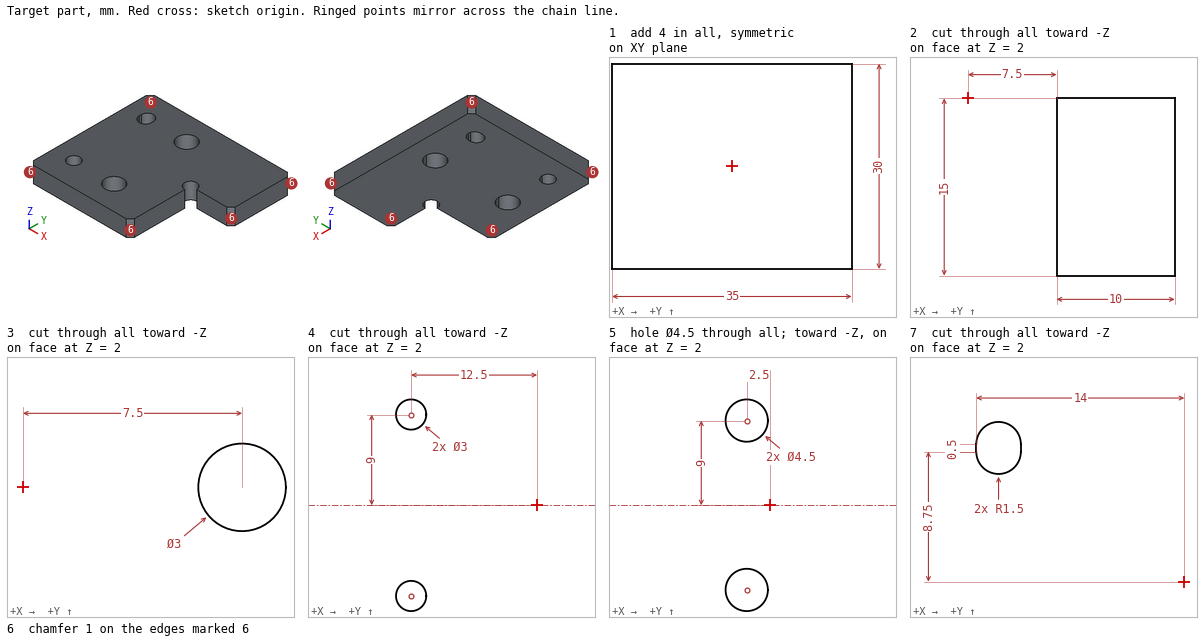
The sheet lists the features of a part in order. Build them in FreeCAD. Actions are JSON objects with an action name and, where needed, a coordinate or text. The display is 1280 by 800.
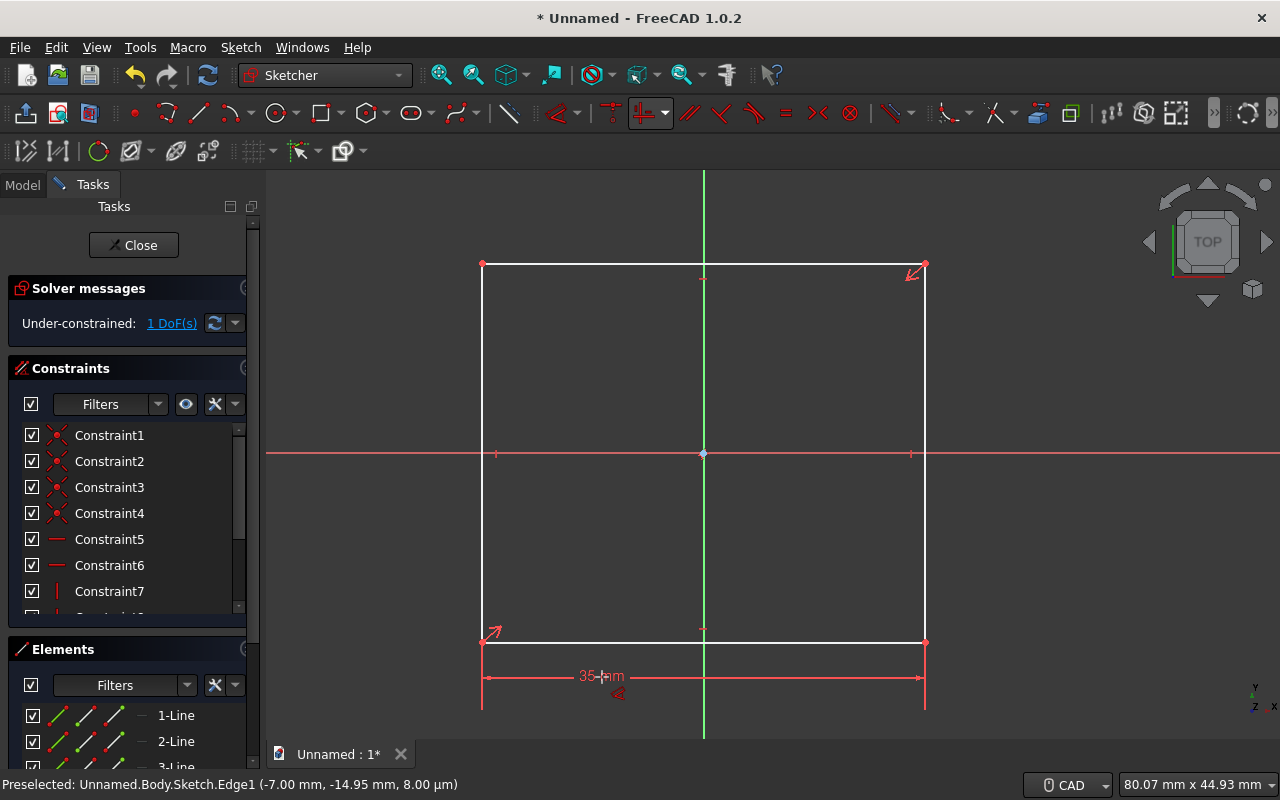
{"action": "left_click", "coordinate": [925, 529]}
{"action": "left_click", "coordinate": [959, 366]}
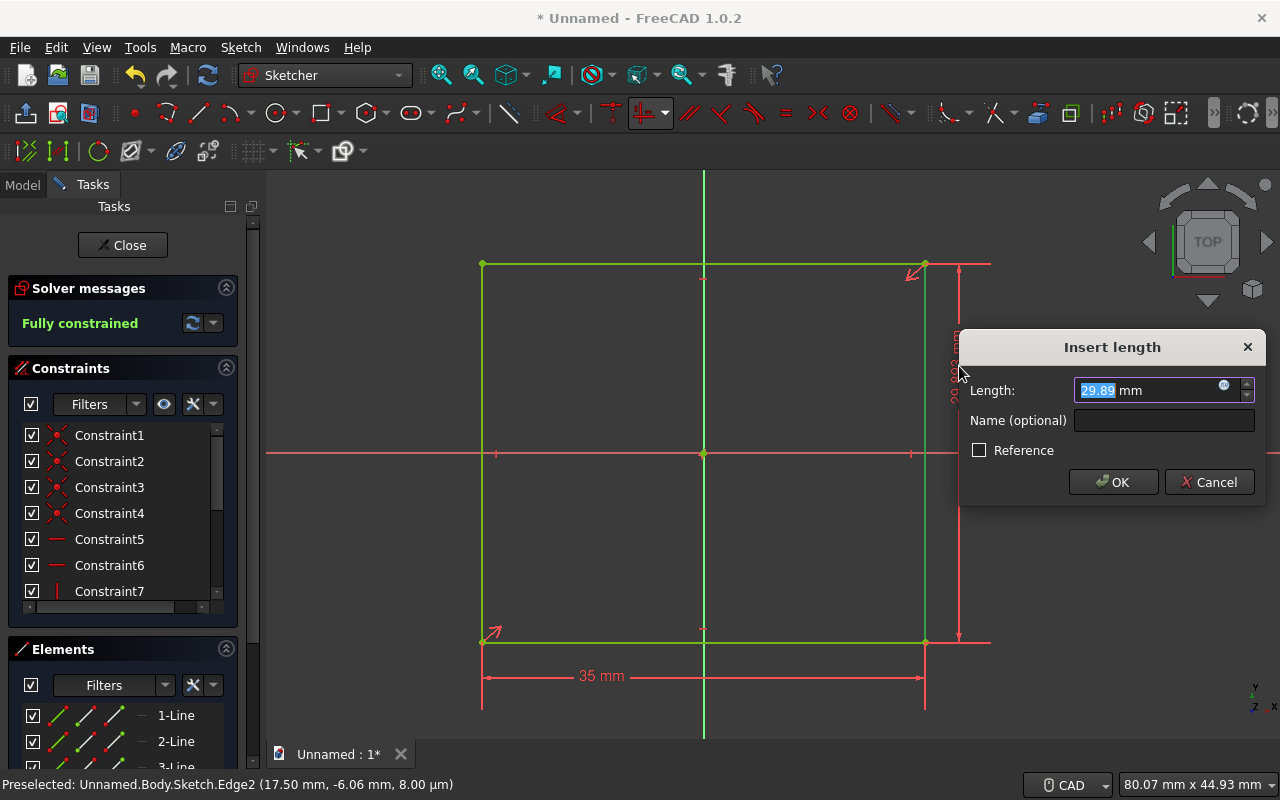
{"action": "type", "text": "30"}
{"action": "key", "text": "Return"}
{"action": "key", "text": "Escape"}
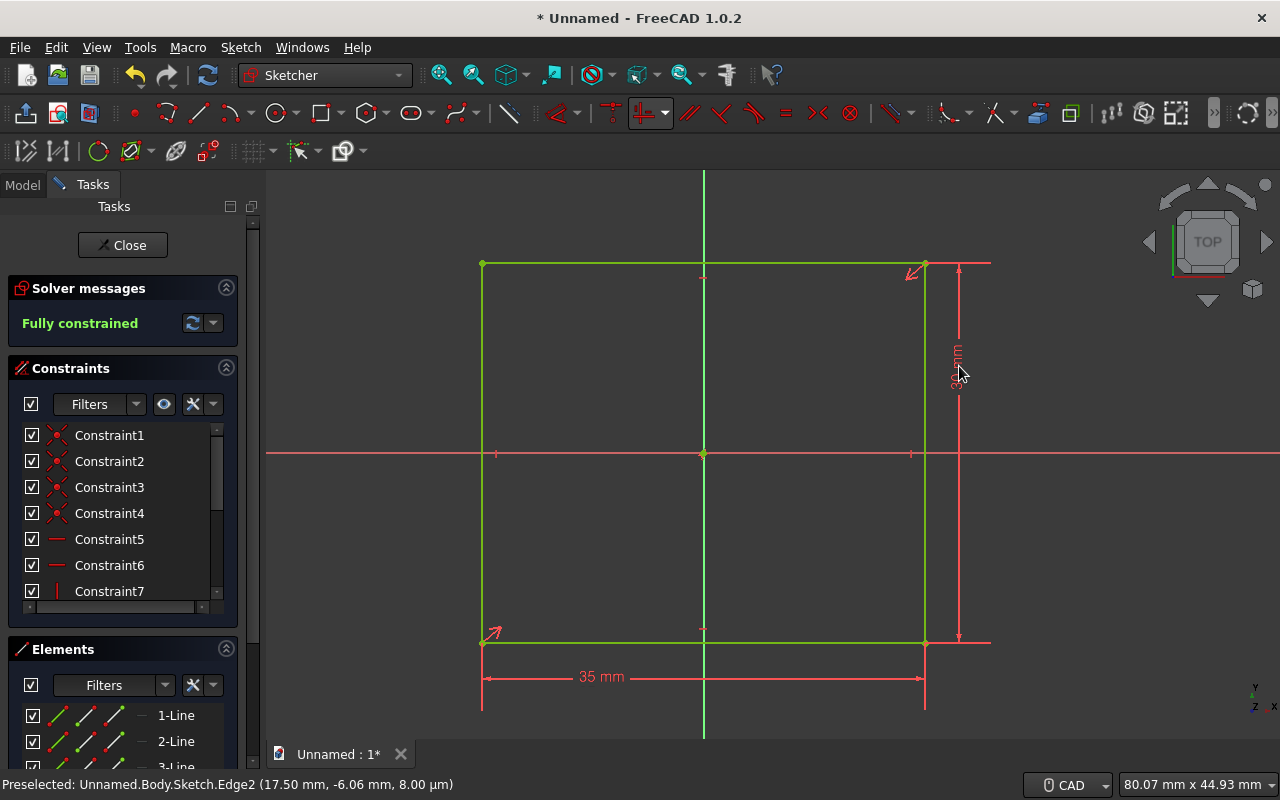
{"action": "left_click", "coordinate": [123, 245]}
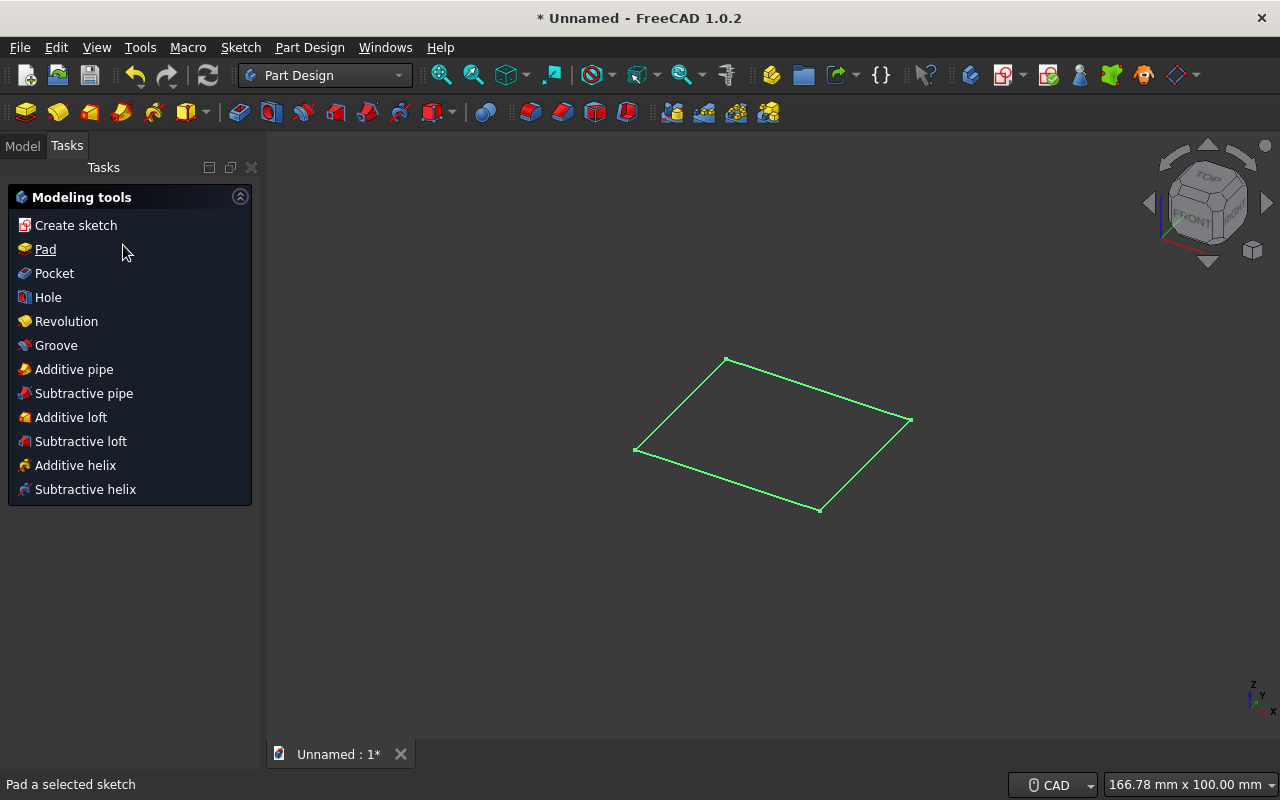
{"action": "left_click", "coordinate": [26, 112]}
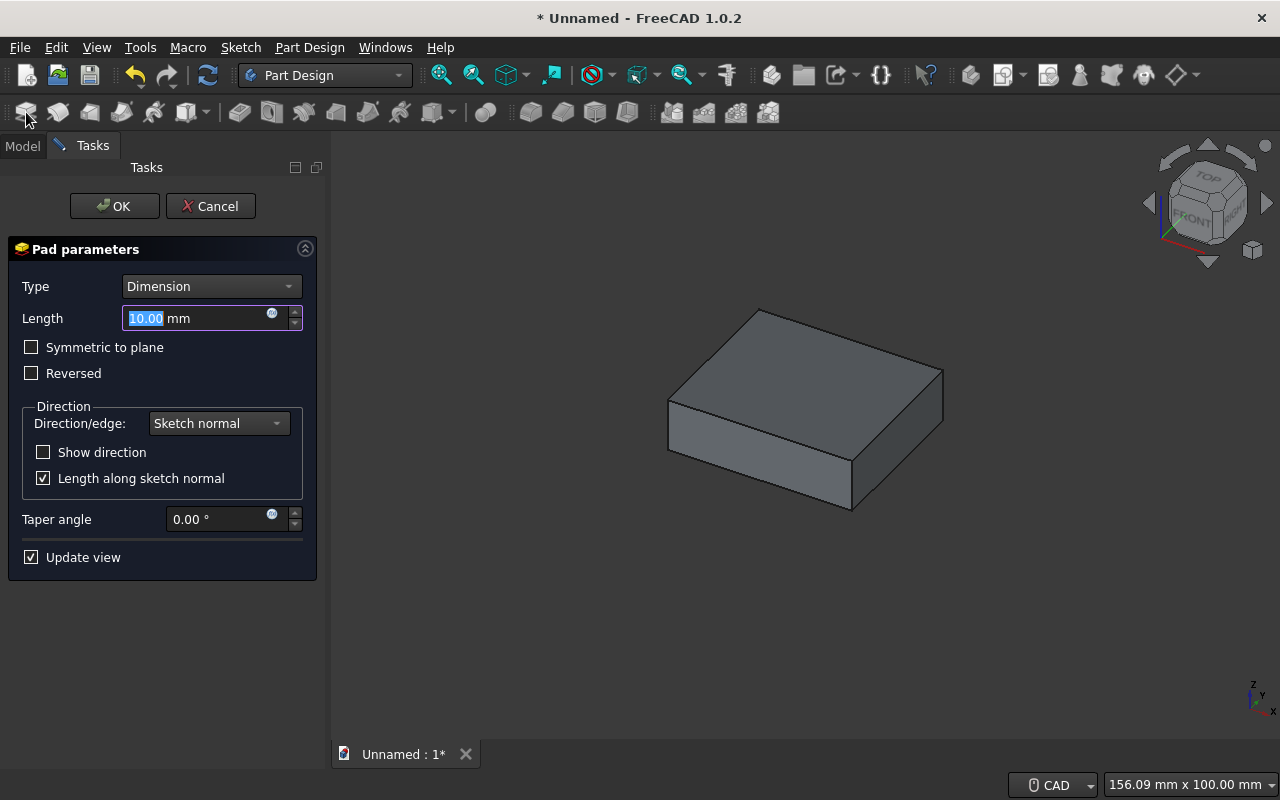
{"action": "type", "text": "4"}
{"action": "key", "text": "Tab"}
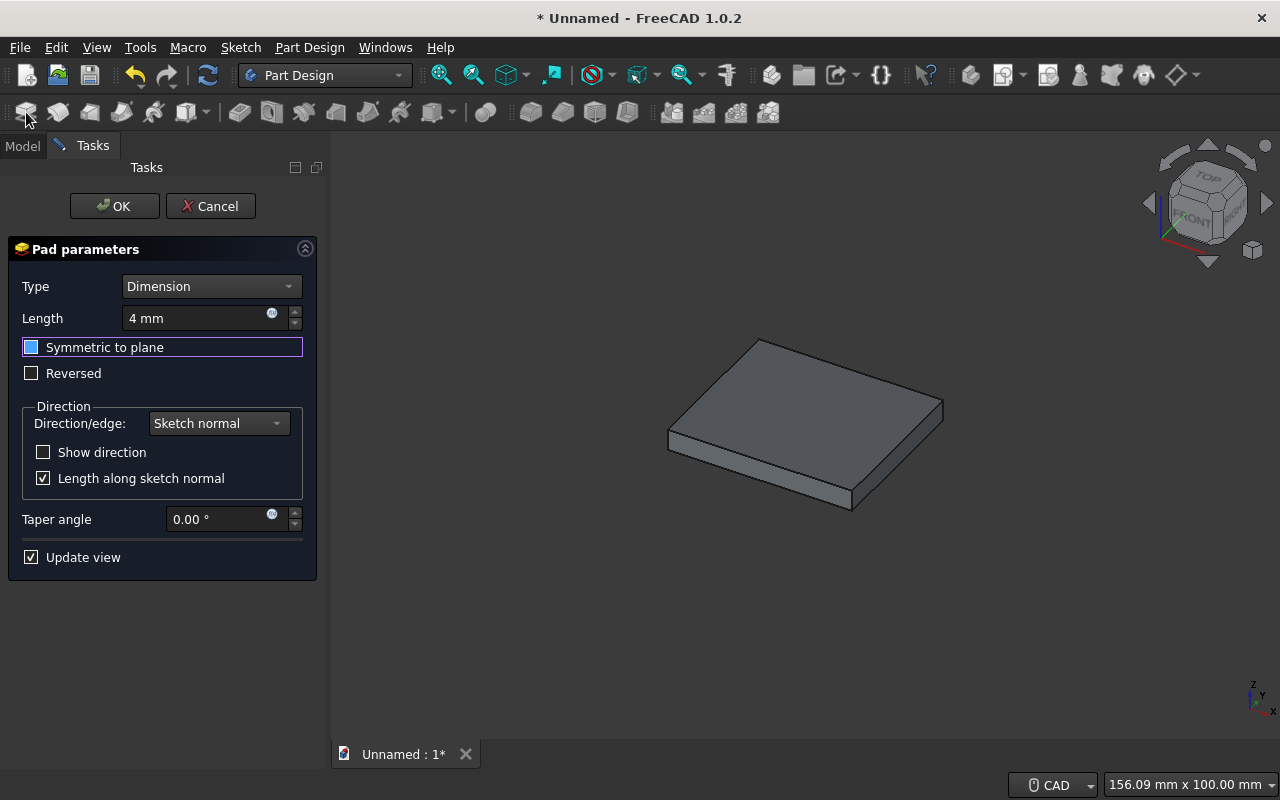
{"action": "left_click", "coordinate": [30, 347]}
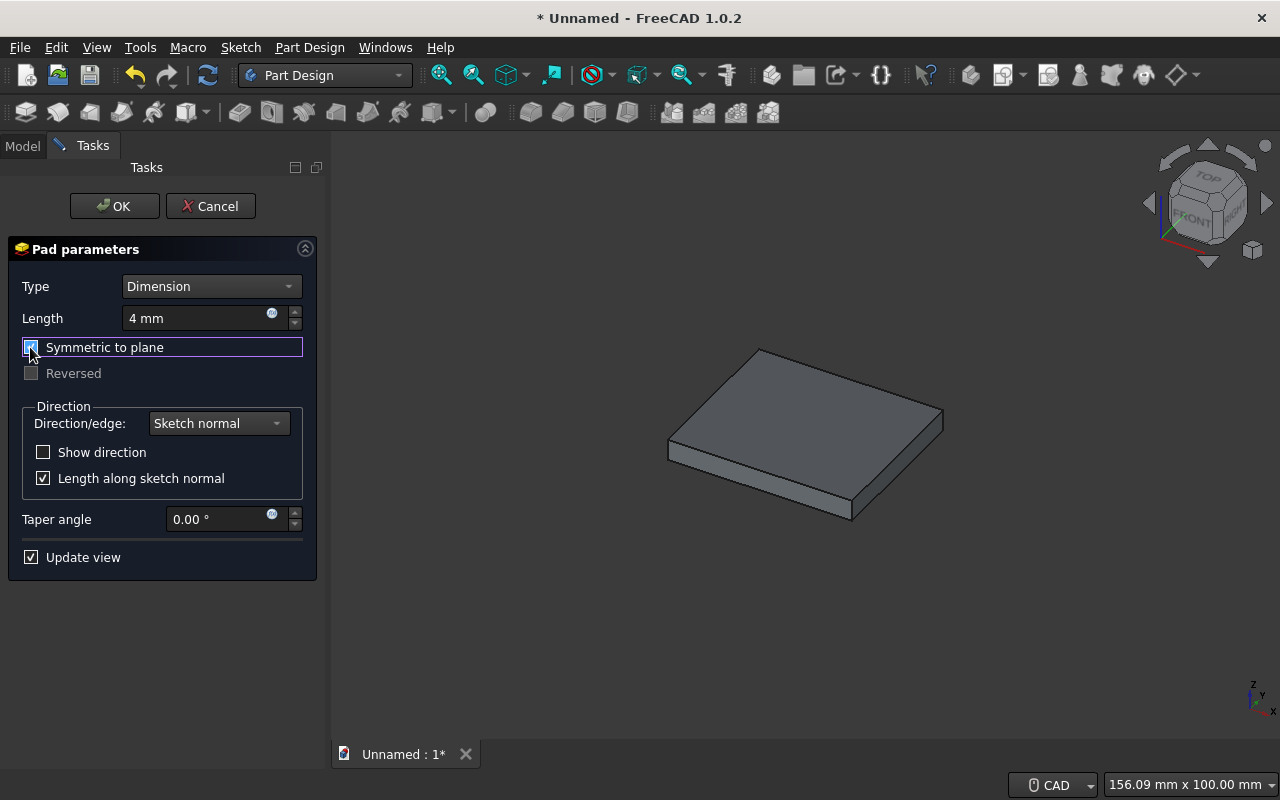
{"action": "left_click", "coordinate": [115, 206]}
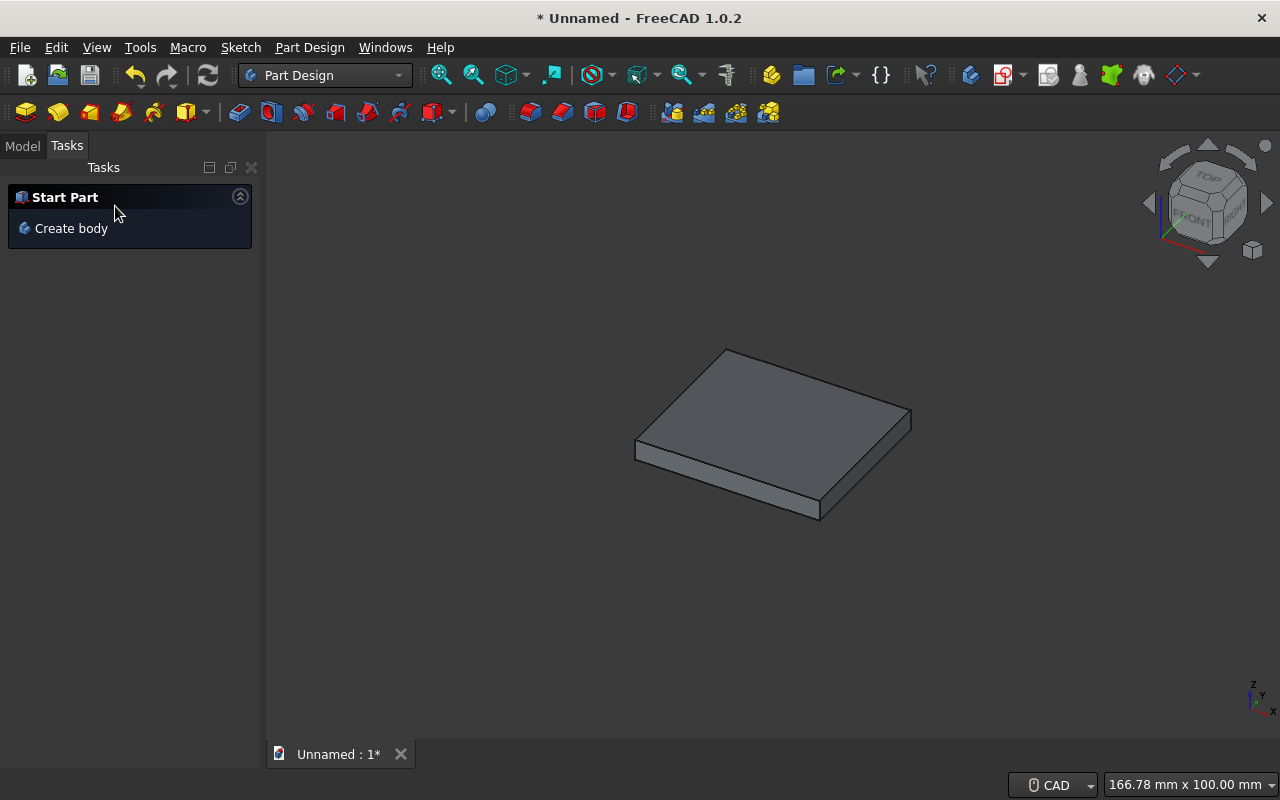
{"action": "key", "text": "v f"}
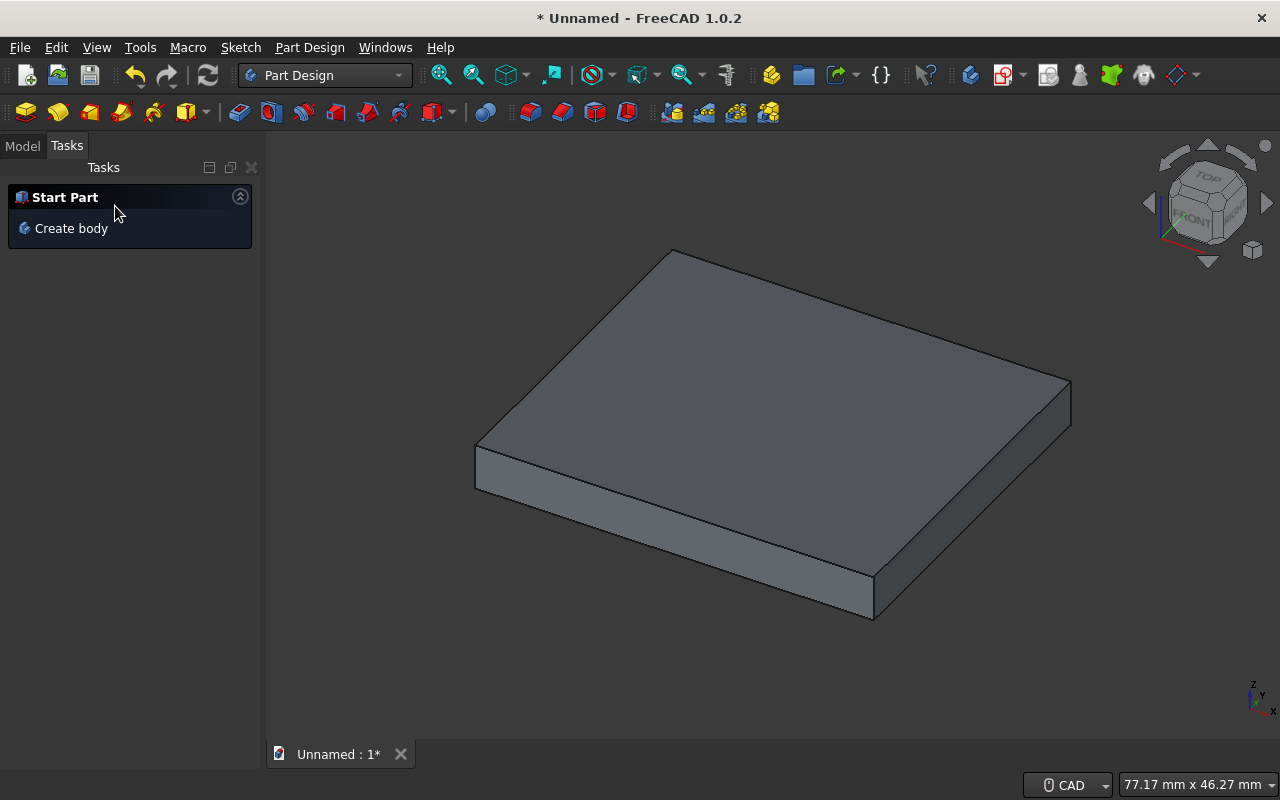
{"action": "left_click", "coordinate": [773, 412]}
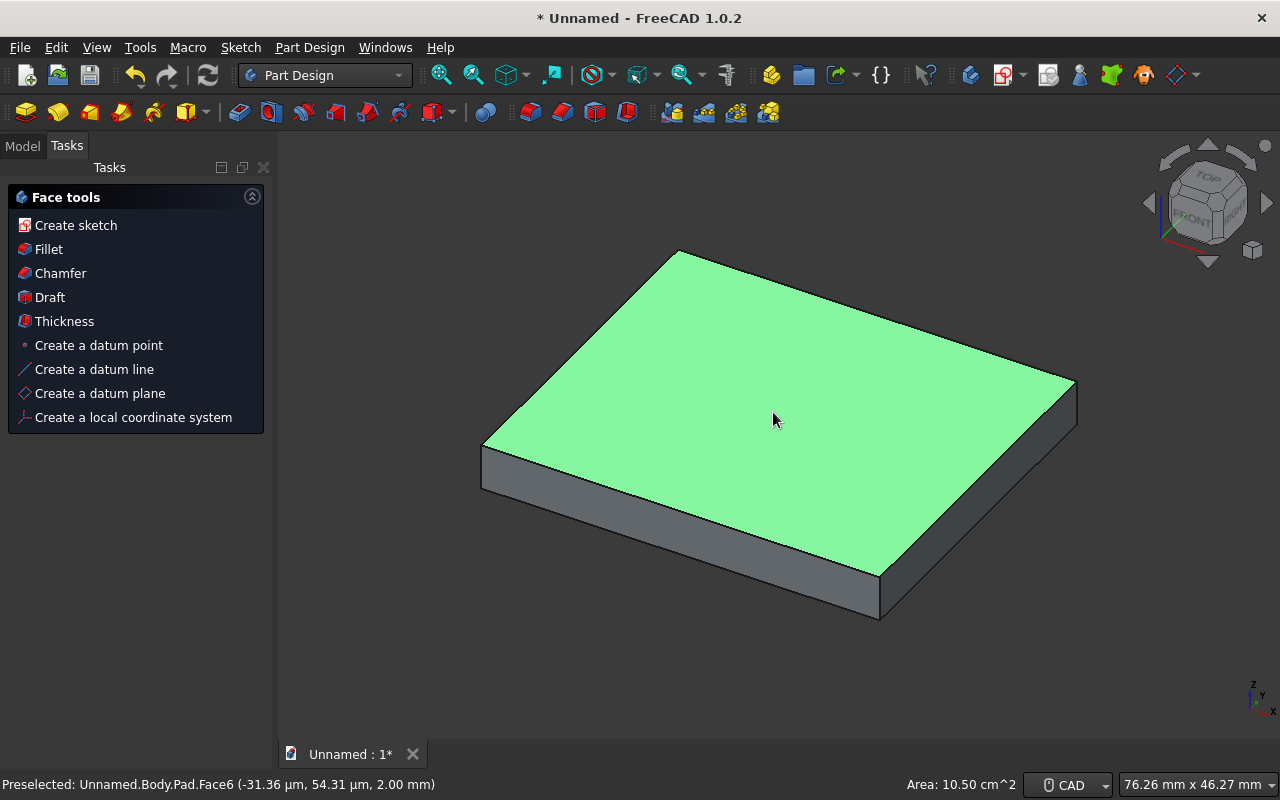
{"action": "left_click", "coordinate": [1004, 76]}